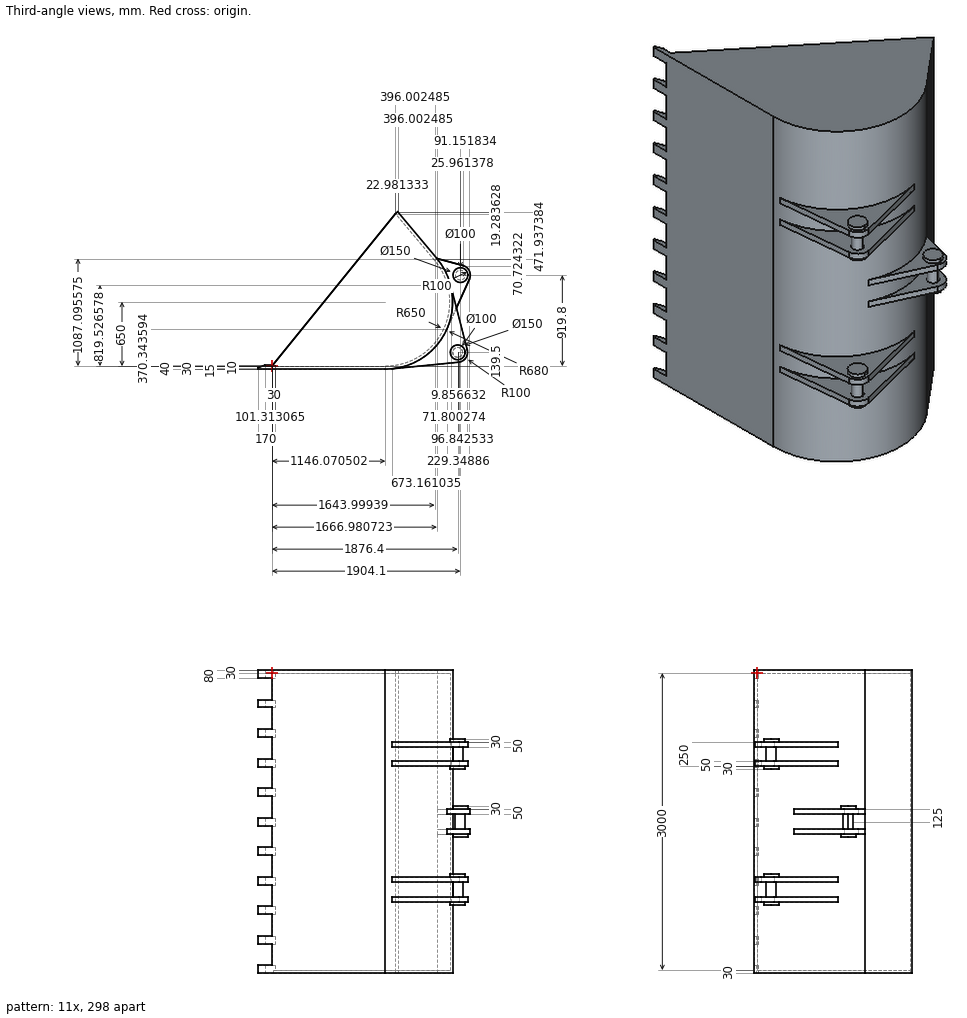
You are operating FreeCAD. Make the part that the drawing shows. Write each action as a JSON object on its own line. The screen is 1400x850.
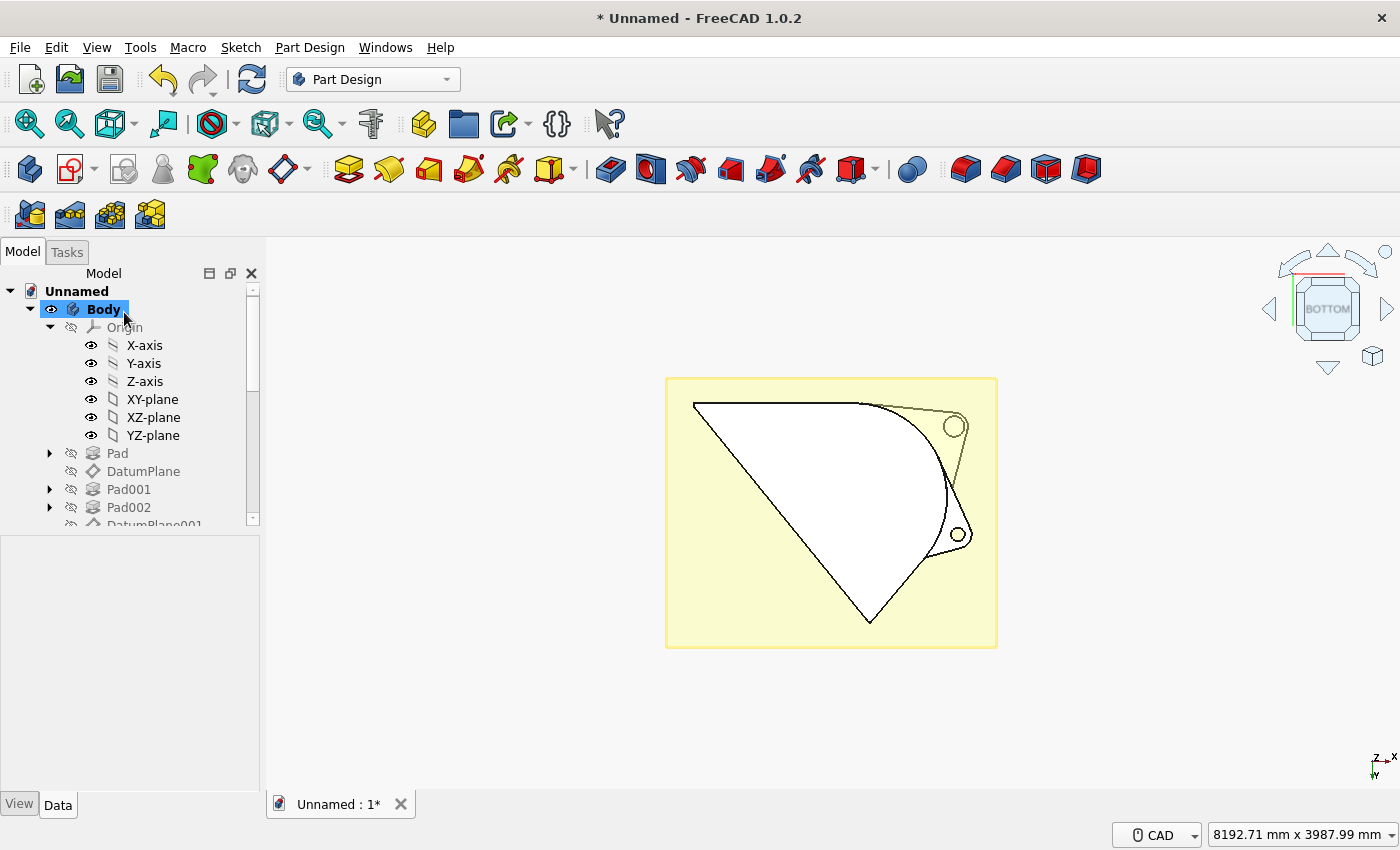
{"action": "scroll", "coordinate": [100, 413], "scroll_direction": "down", "scroll_amount": 3}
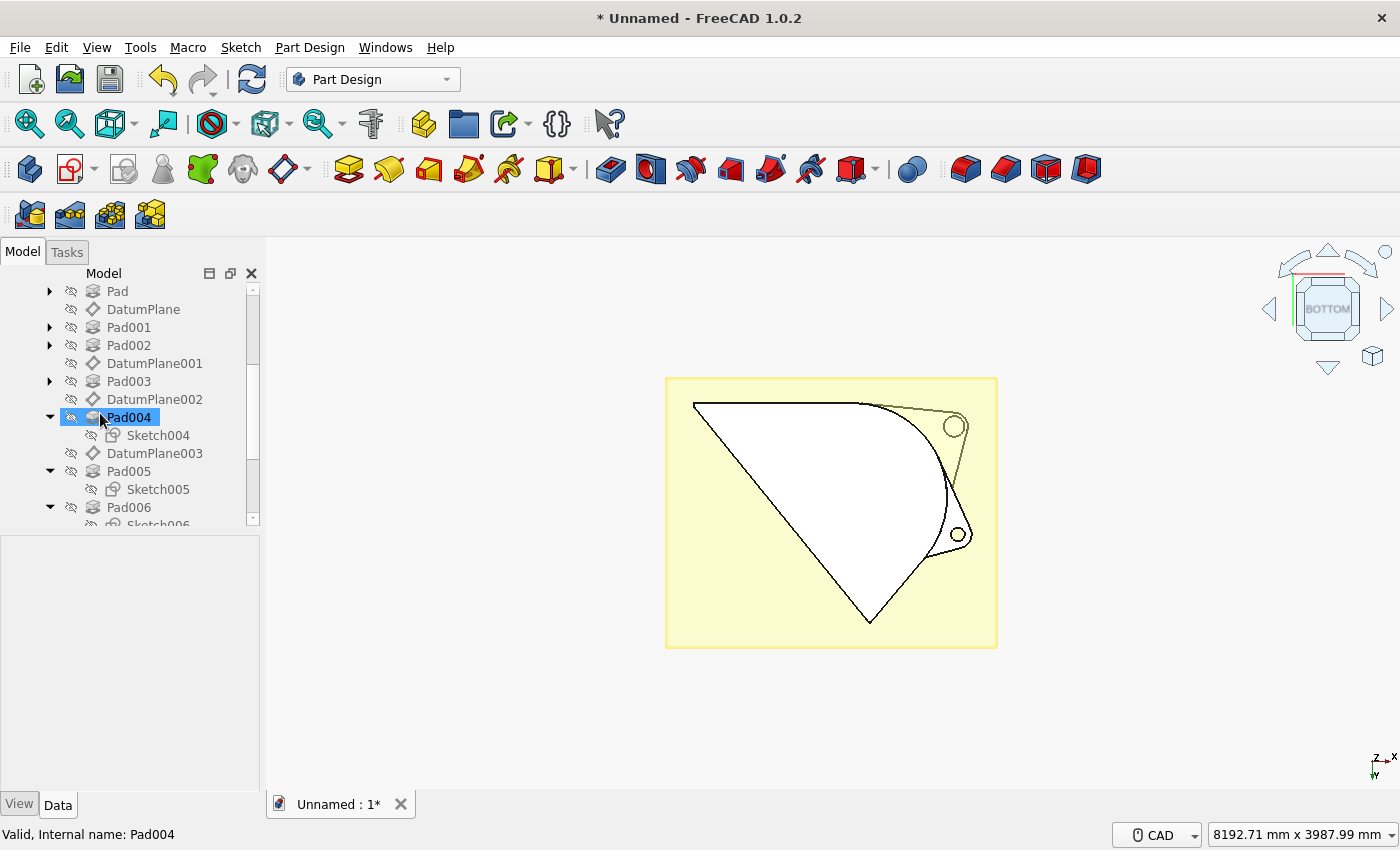
{"action": "scroll", "coordinate": [140, 413], "scroll_direction": "up", "scroll_amount": 15}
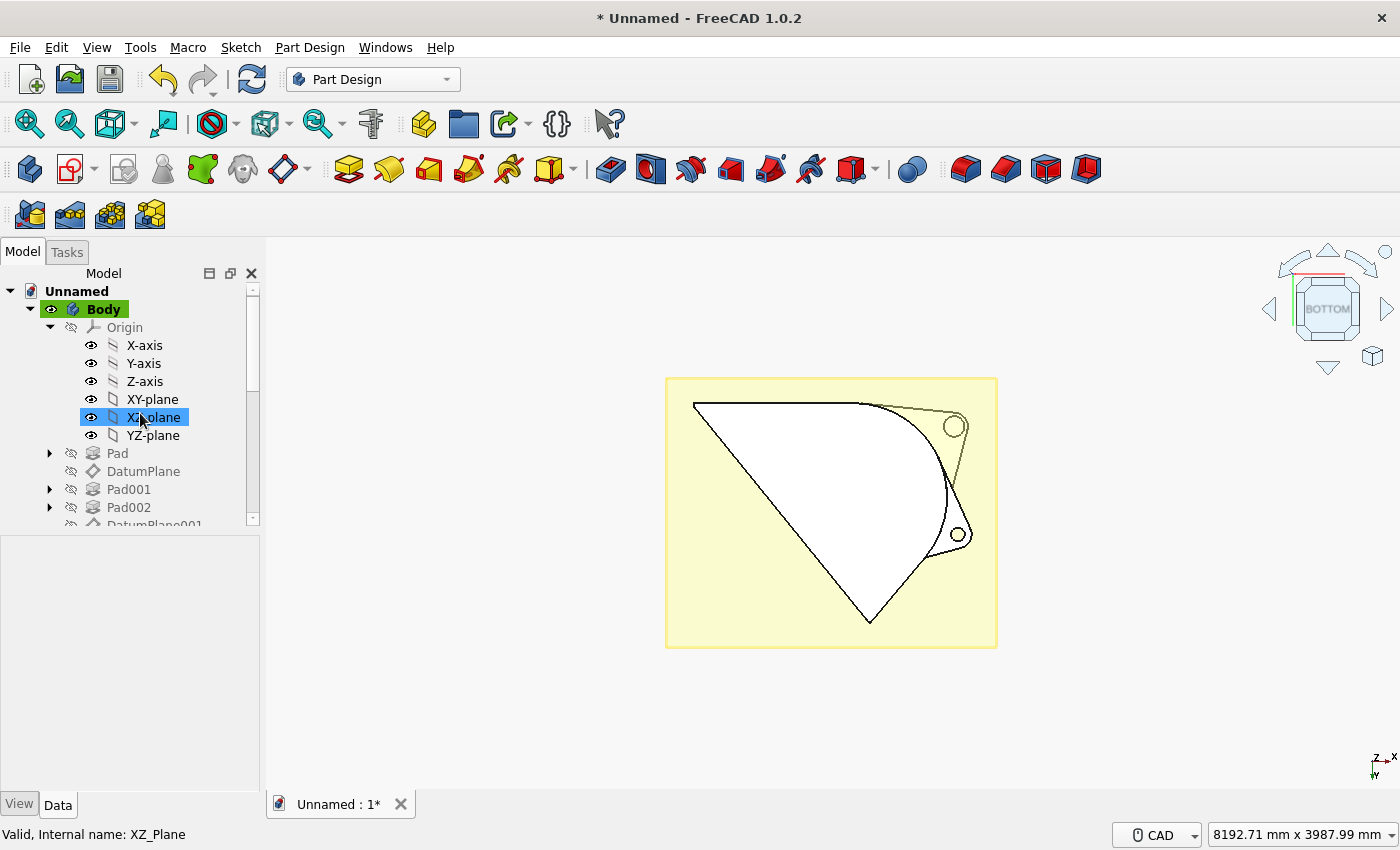
{"action": "scroll", "coordinate": [100, 413], "scroll_direction": "down", "scroll_amount": 6}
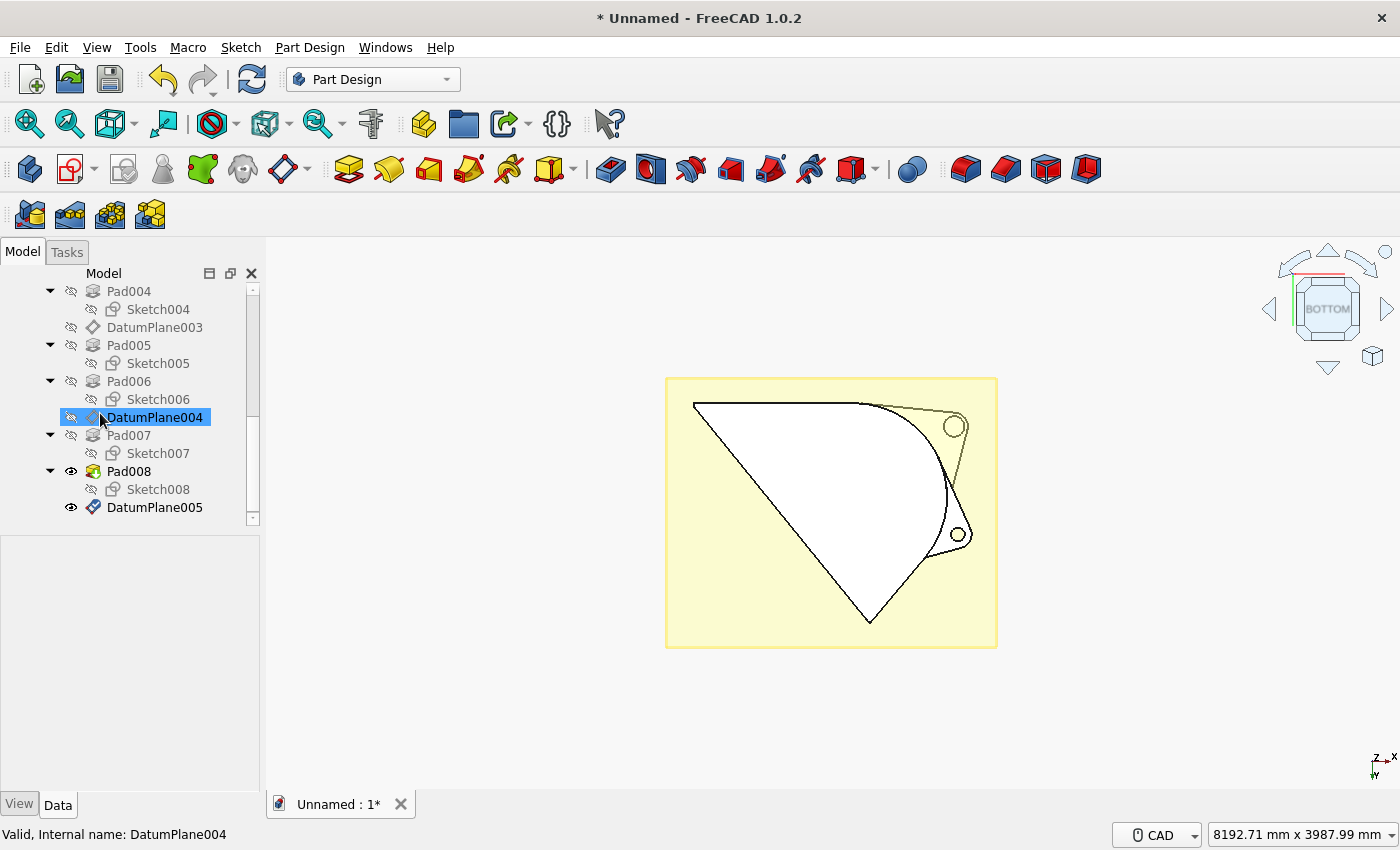
{"action": "left_click", "coordinate": [116, 507]}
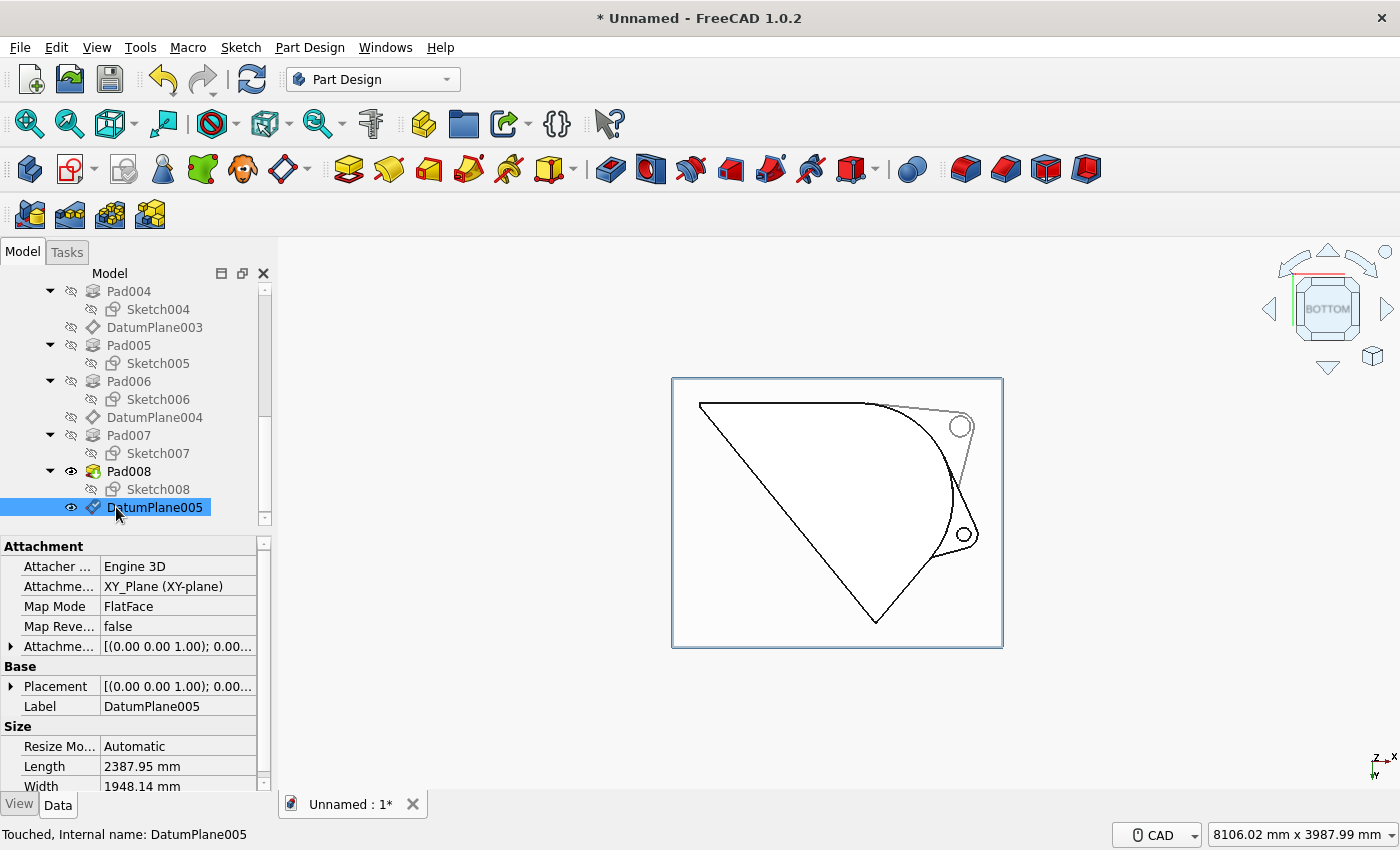
{"action": "left_click", "coordinate": [70, 170]}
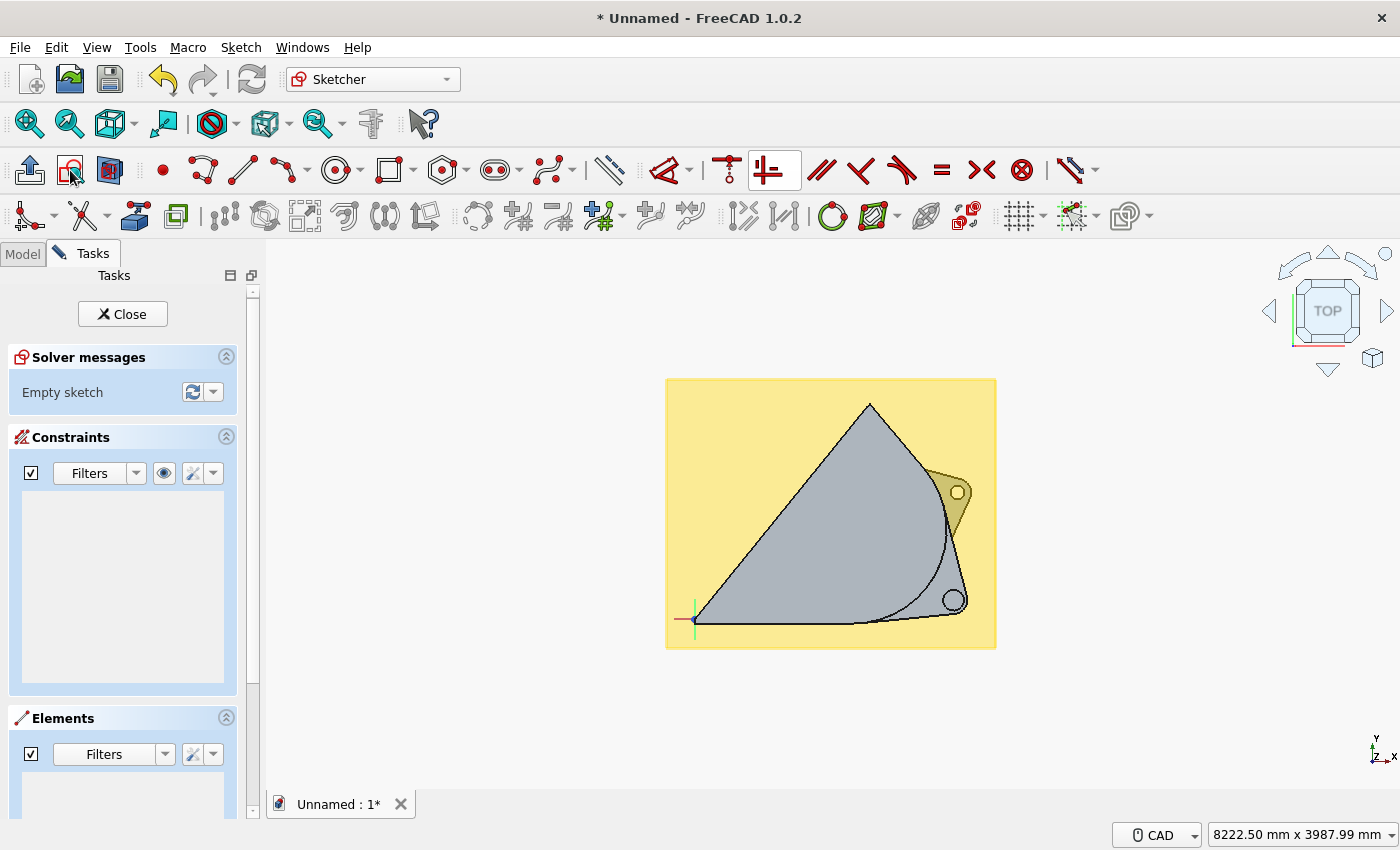
{"action": "left_click", "coordinate": [110, 170]}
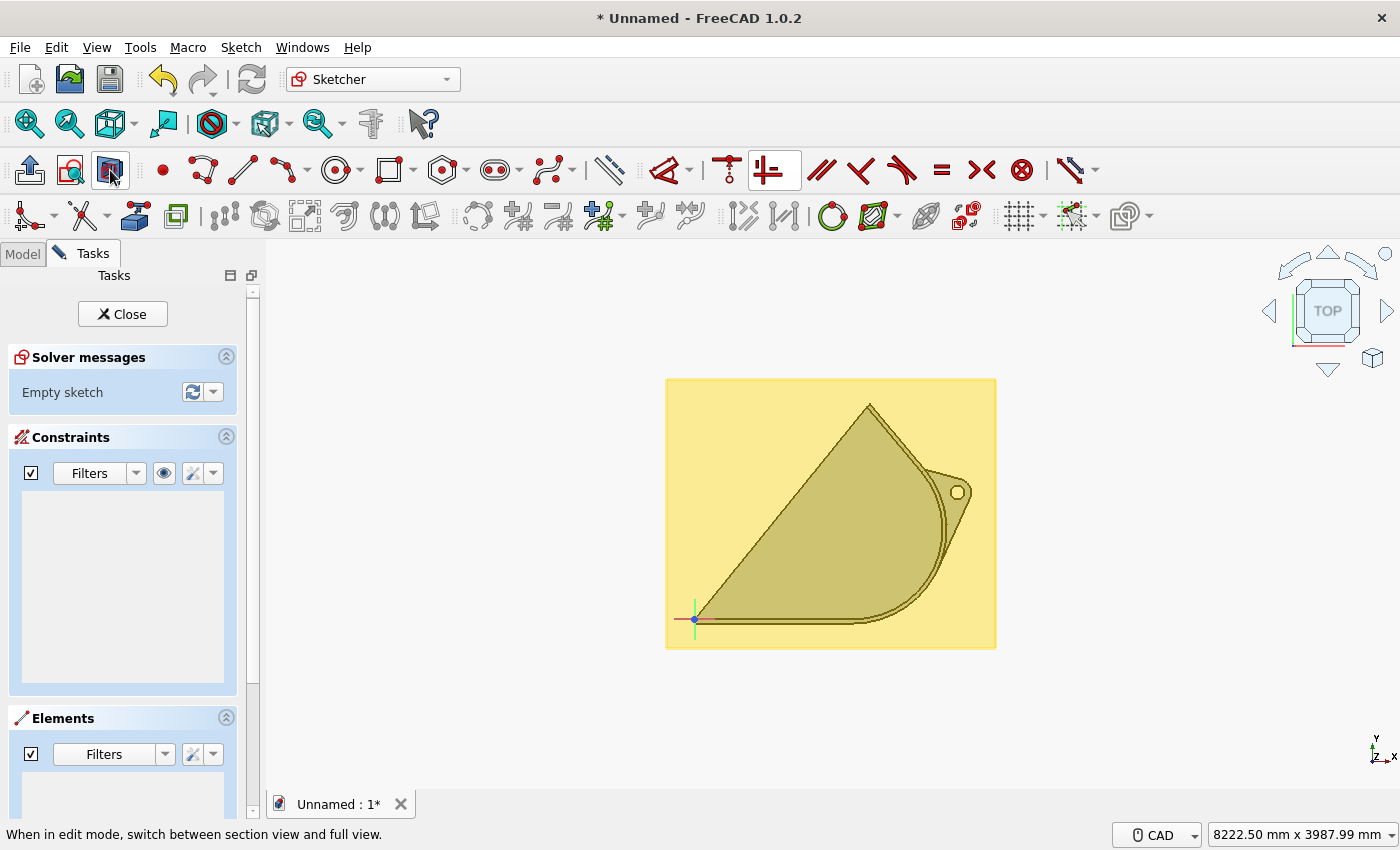
{"action": "scroll", "coordinate": [970, 491], "scroll_direction": "up", "scroll_amount": 14}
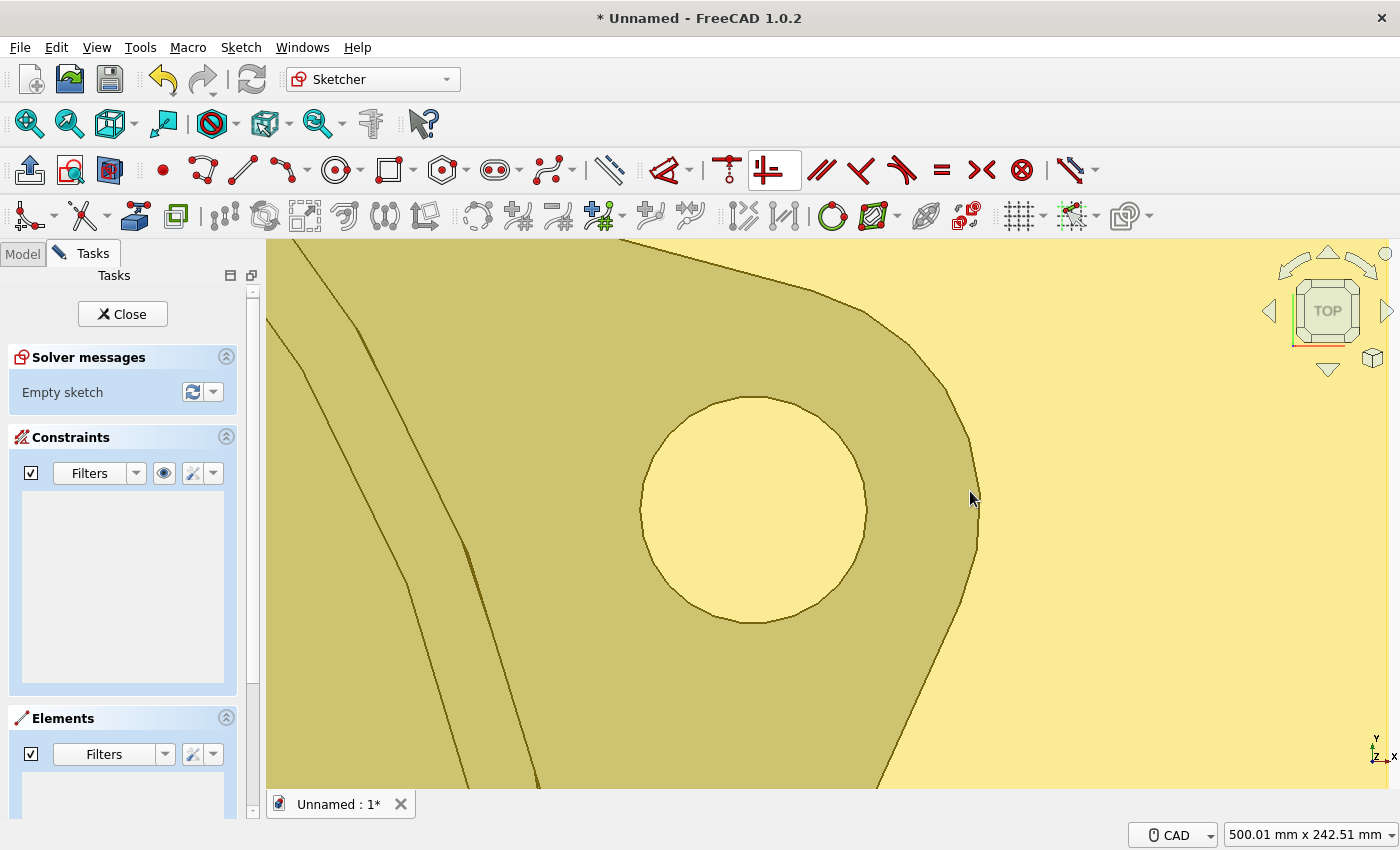
{"action": "left_click", "coordinate": [336, 170]}